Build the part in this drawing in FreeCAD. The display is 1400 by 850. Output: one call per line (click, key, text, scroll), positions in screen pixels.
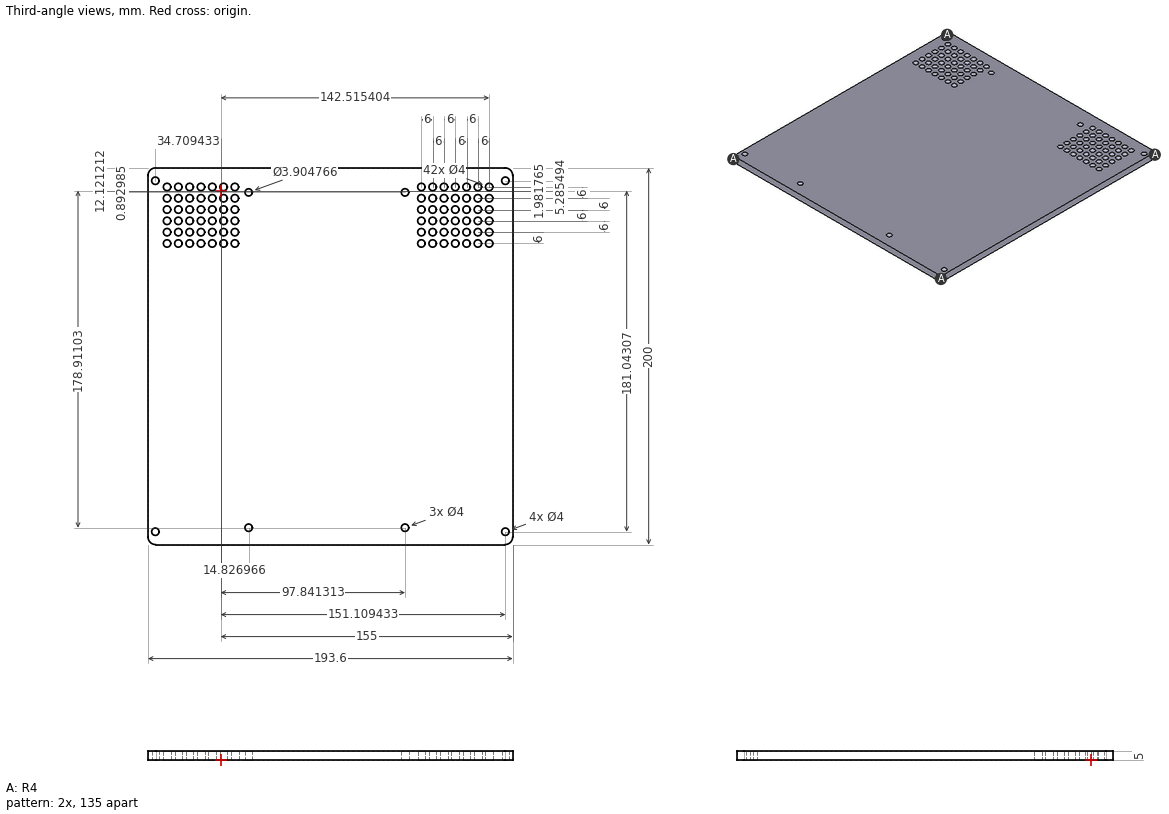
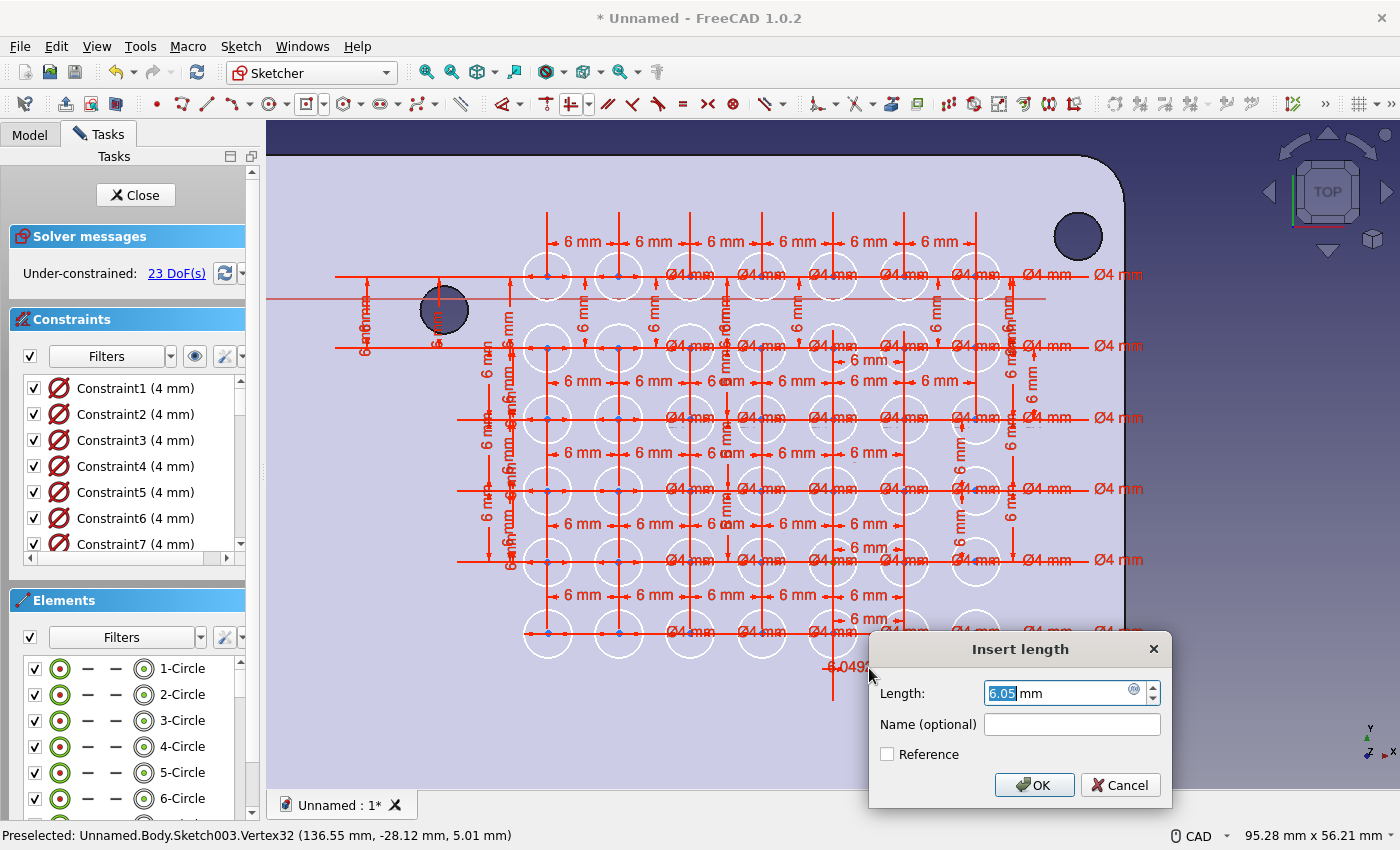
text(6)
key(Return)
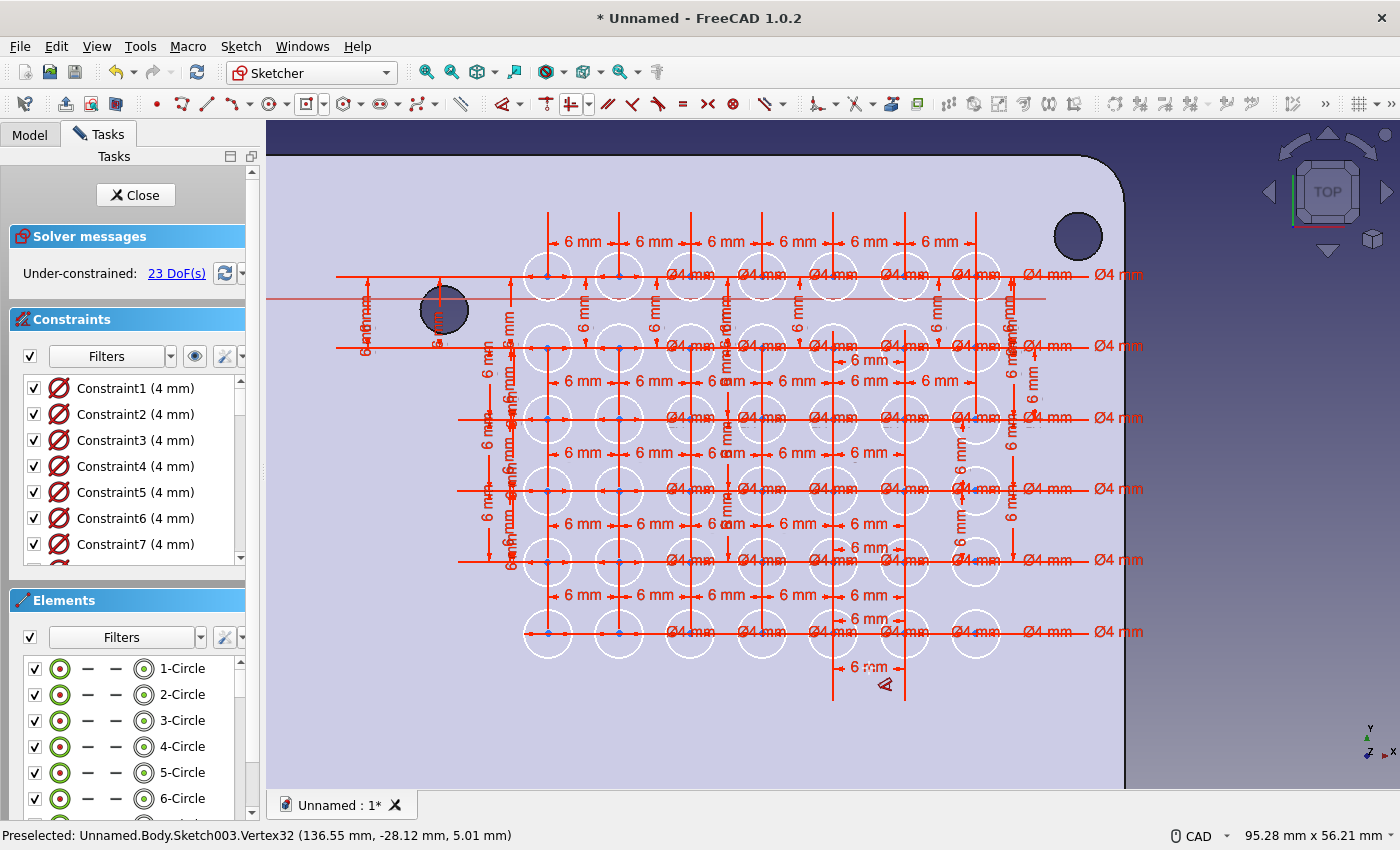
click(905, 562)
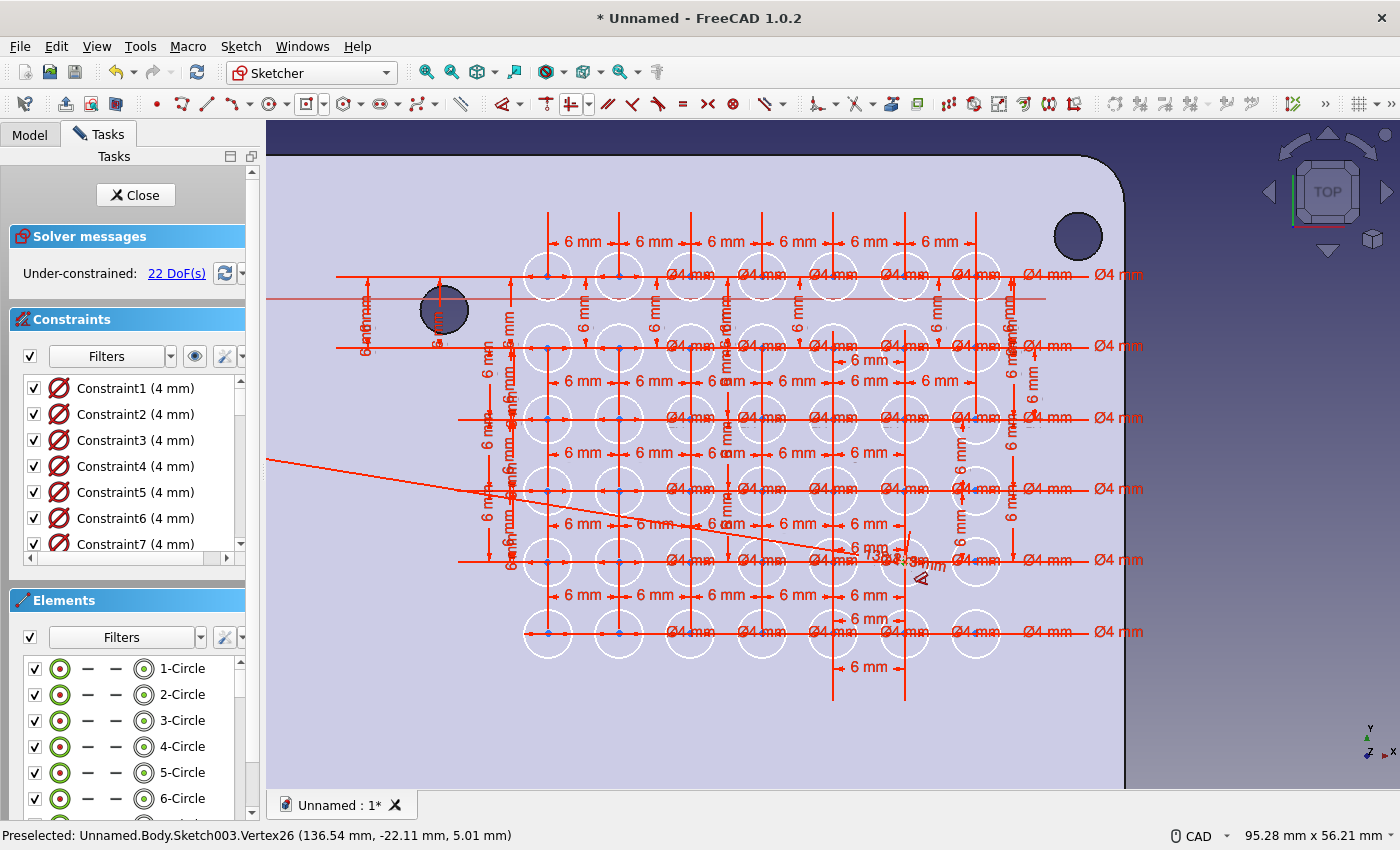
click(905, 634)
click(963, 598)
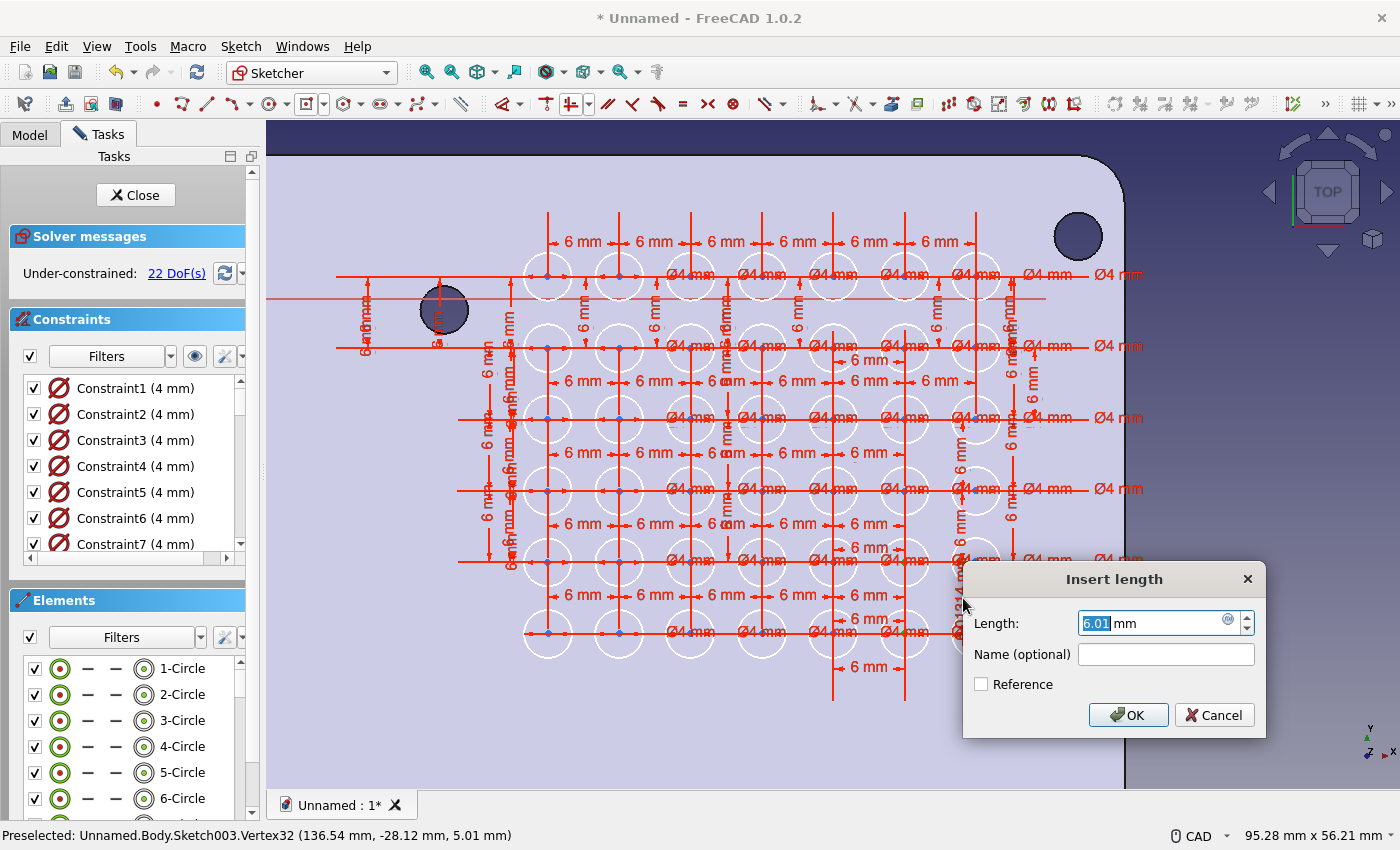
text(6)
key(Return)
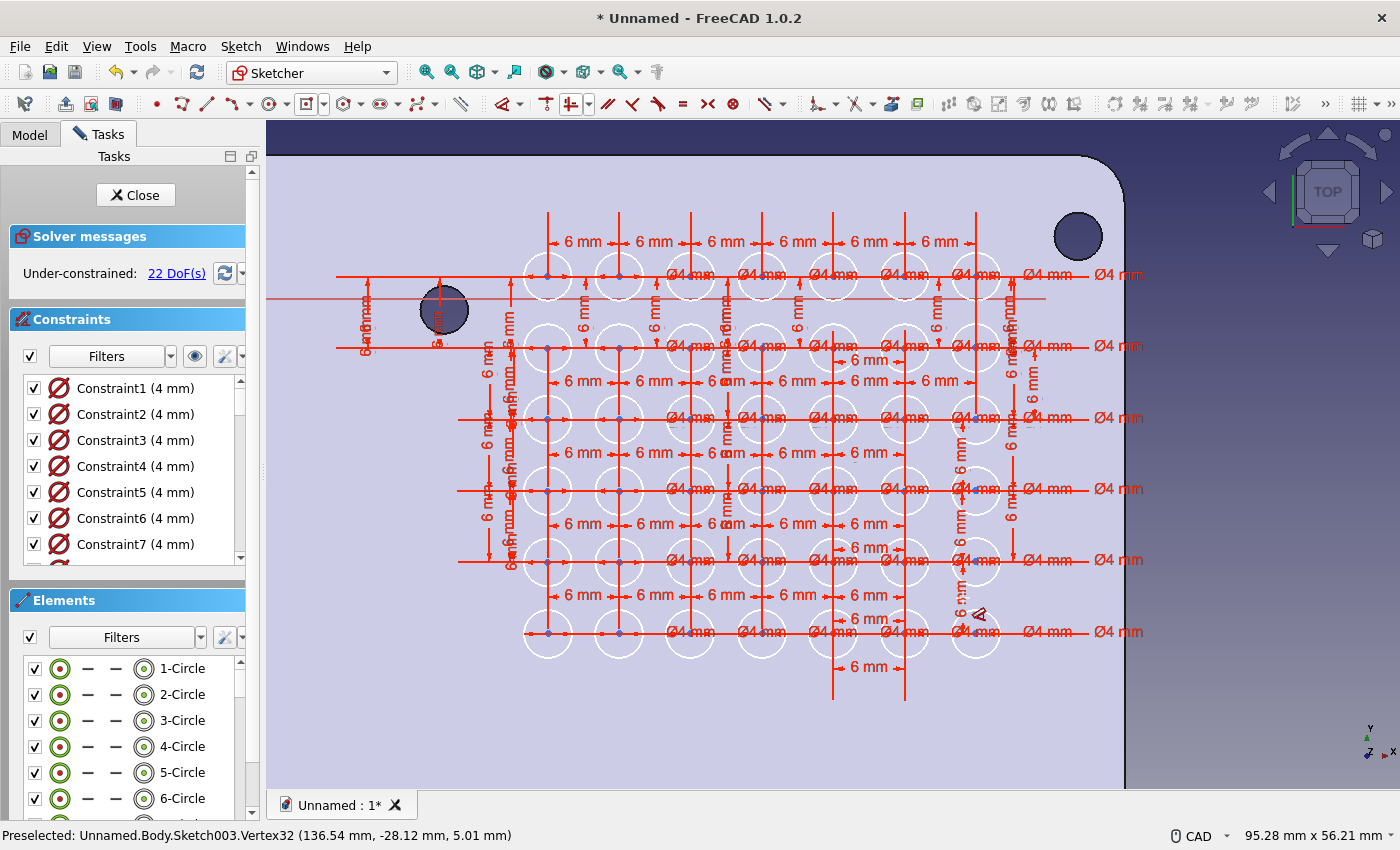
click(905, 634)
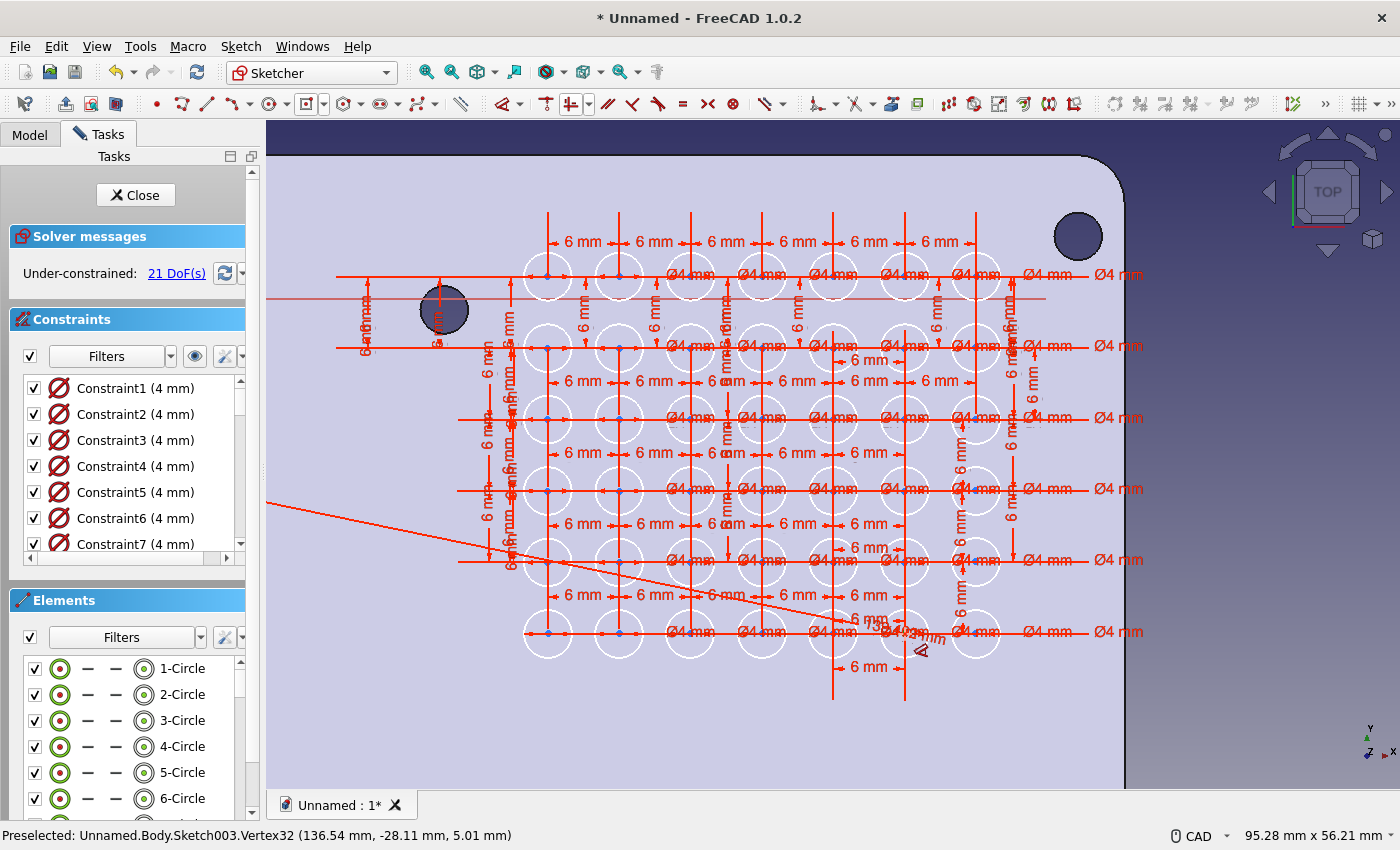
click(833, 634)
click(869, 692)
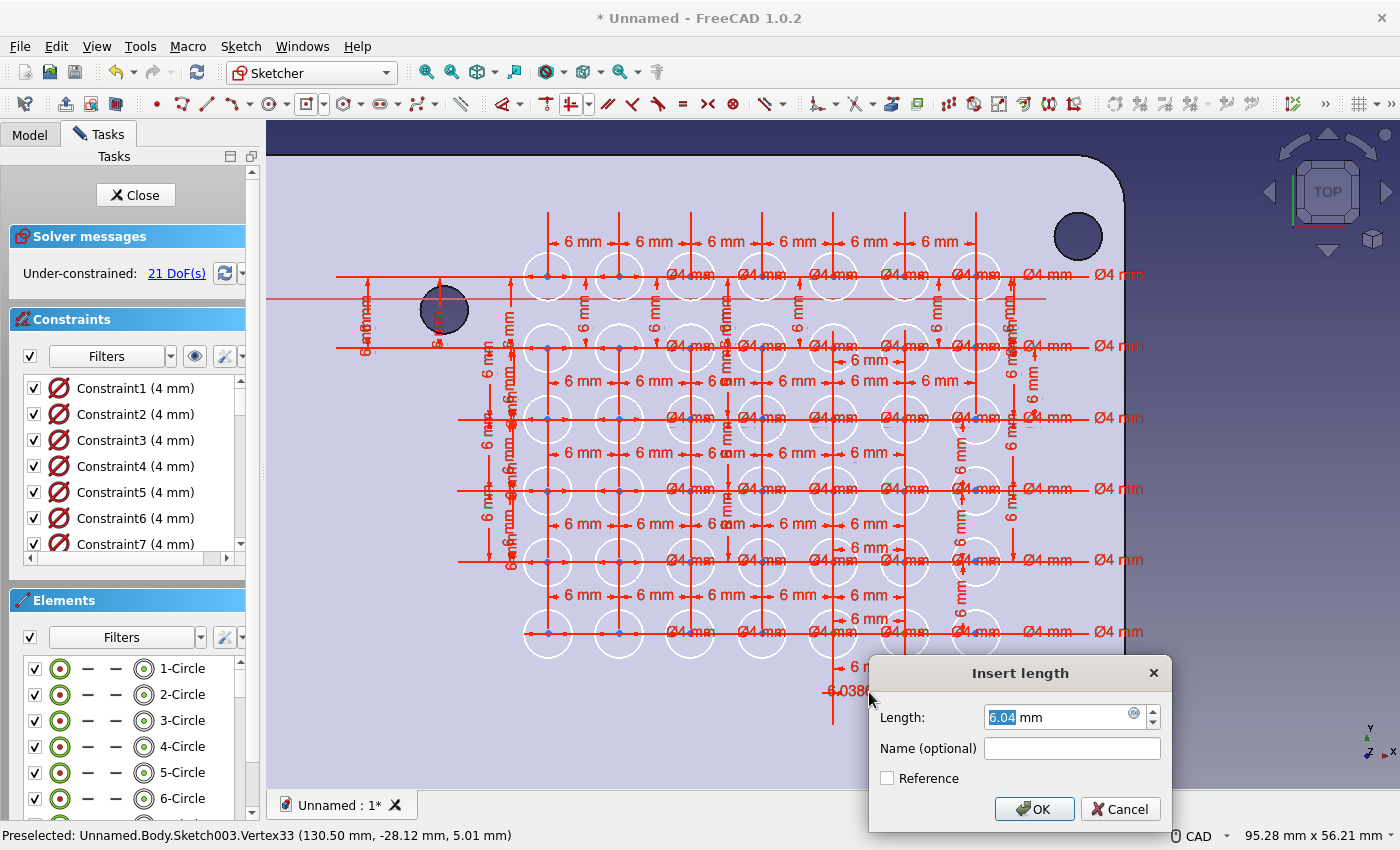
text(6)
key(Return)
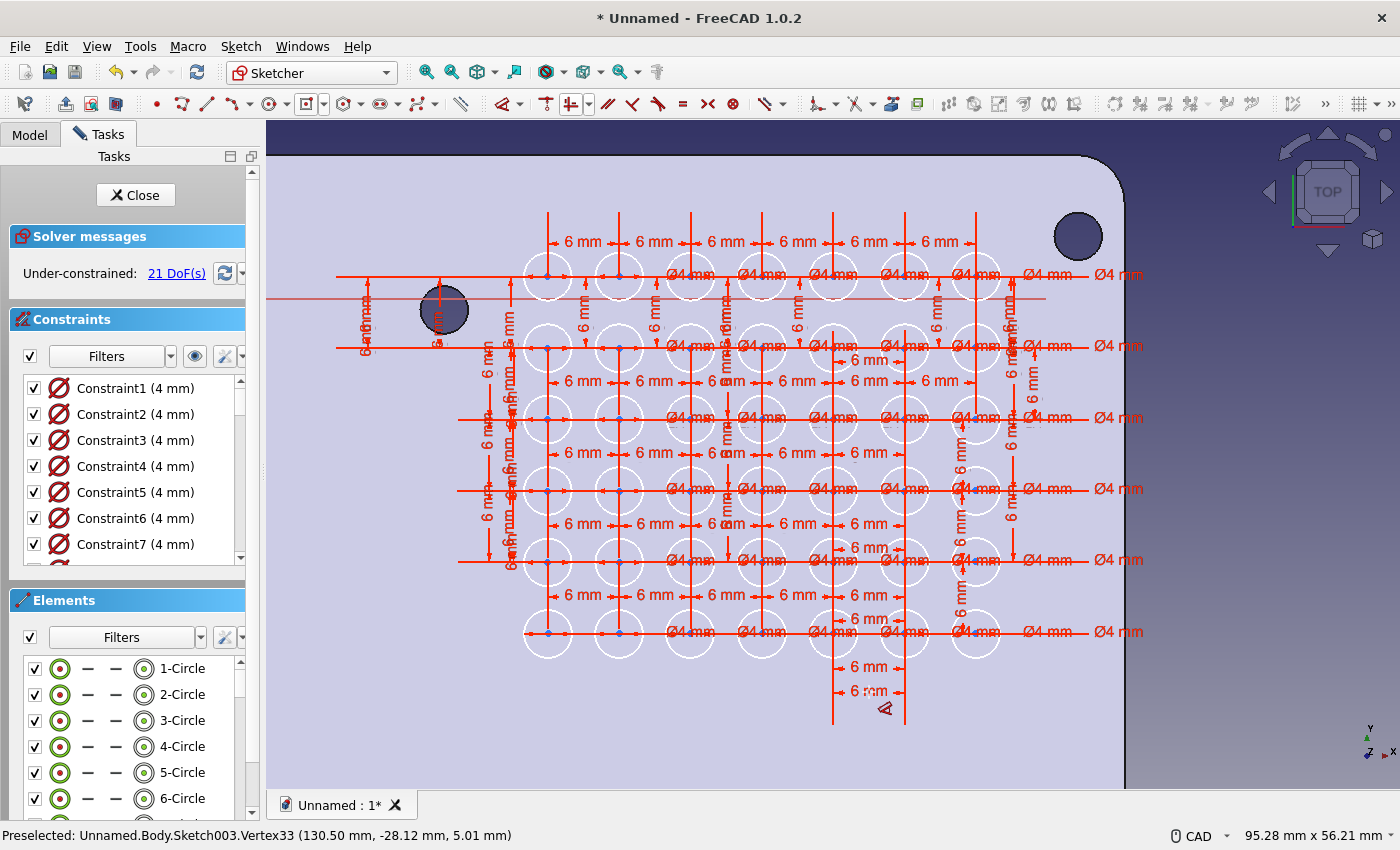
click(833, 562)